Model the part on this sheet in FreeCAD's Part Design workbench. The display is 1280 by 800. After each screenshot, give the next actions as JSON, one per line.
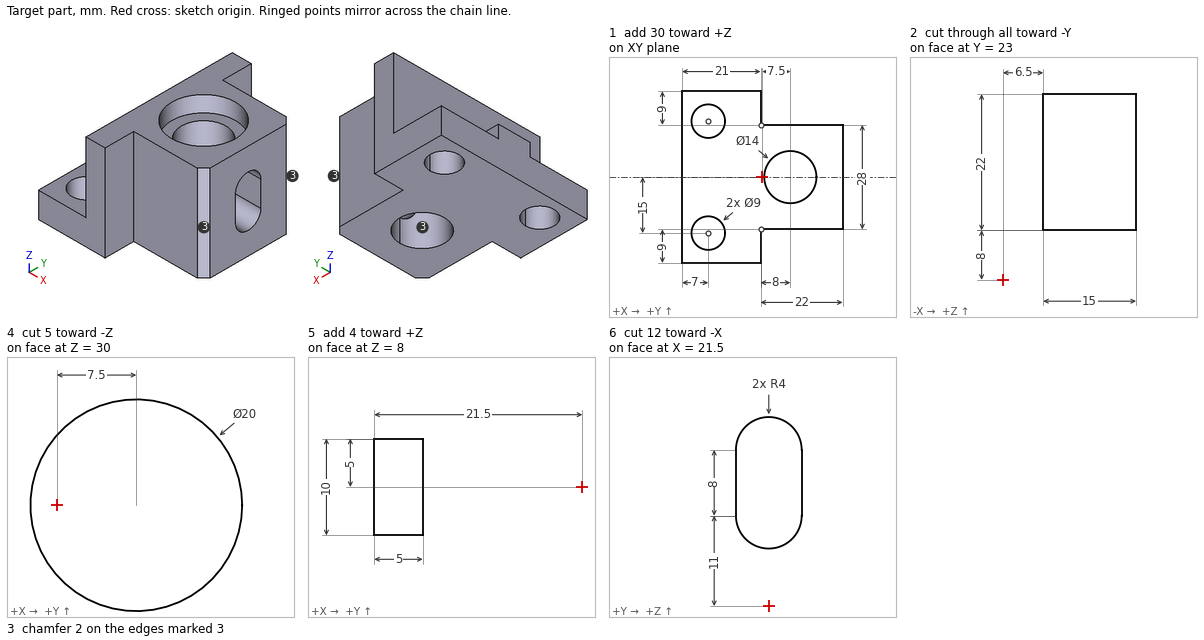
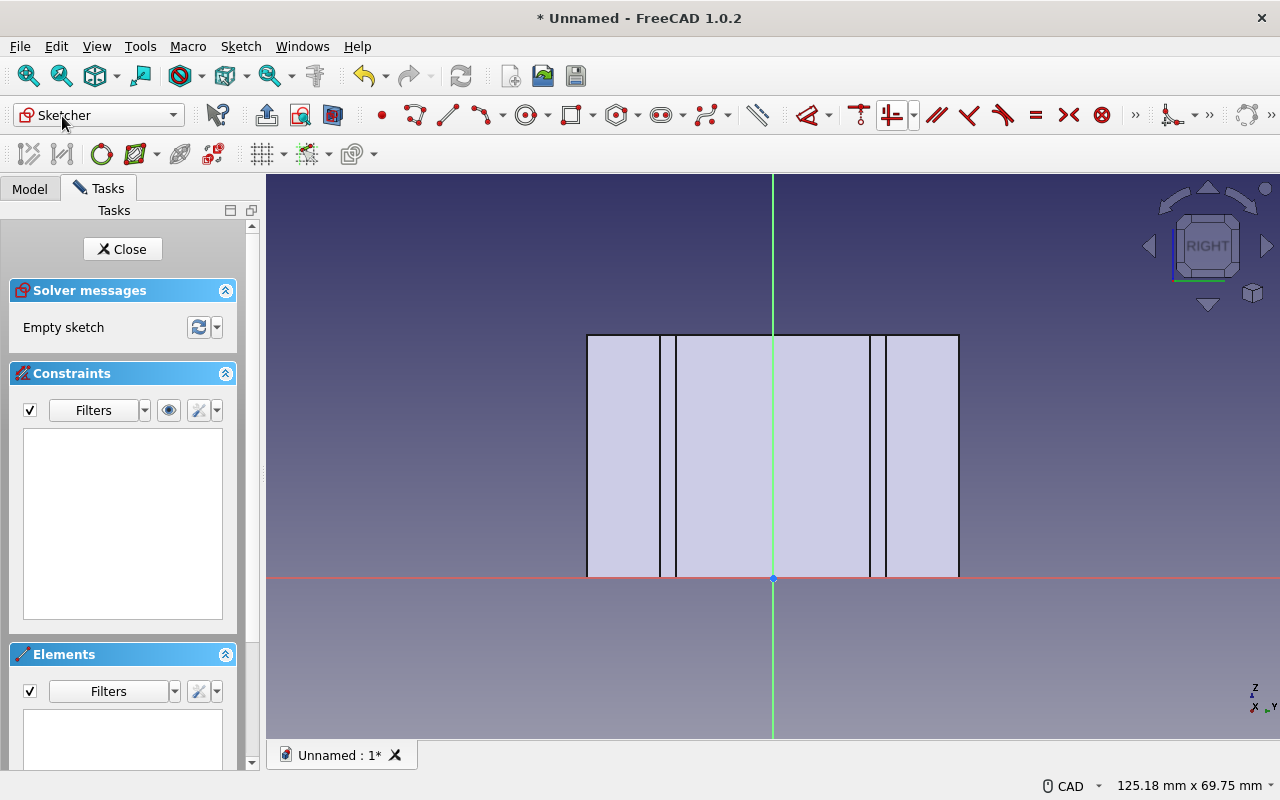
{"action": "scroll", "coordinate": [856, 519], "scroll_direction": "up", "scroll_amount": 3}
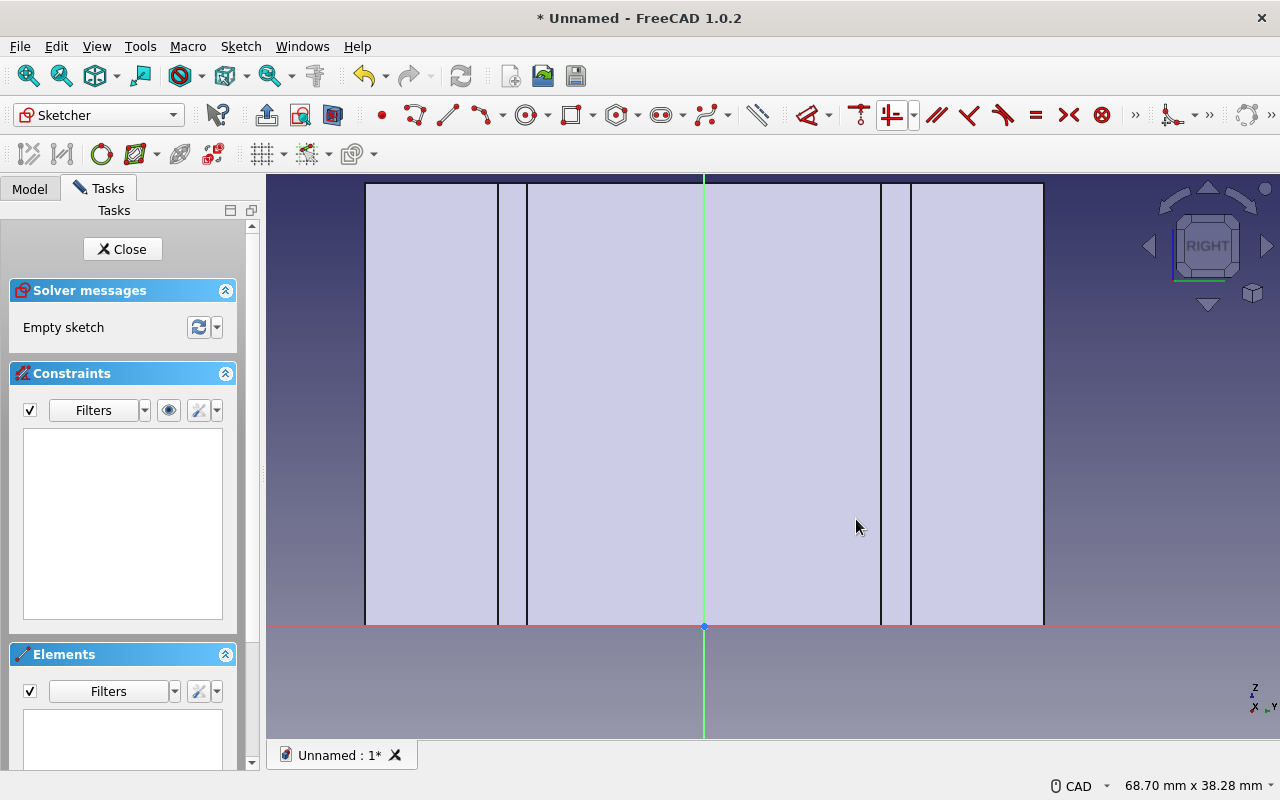
{"action": "key", "text": "g s"}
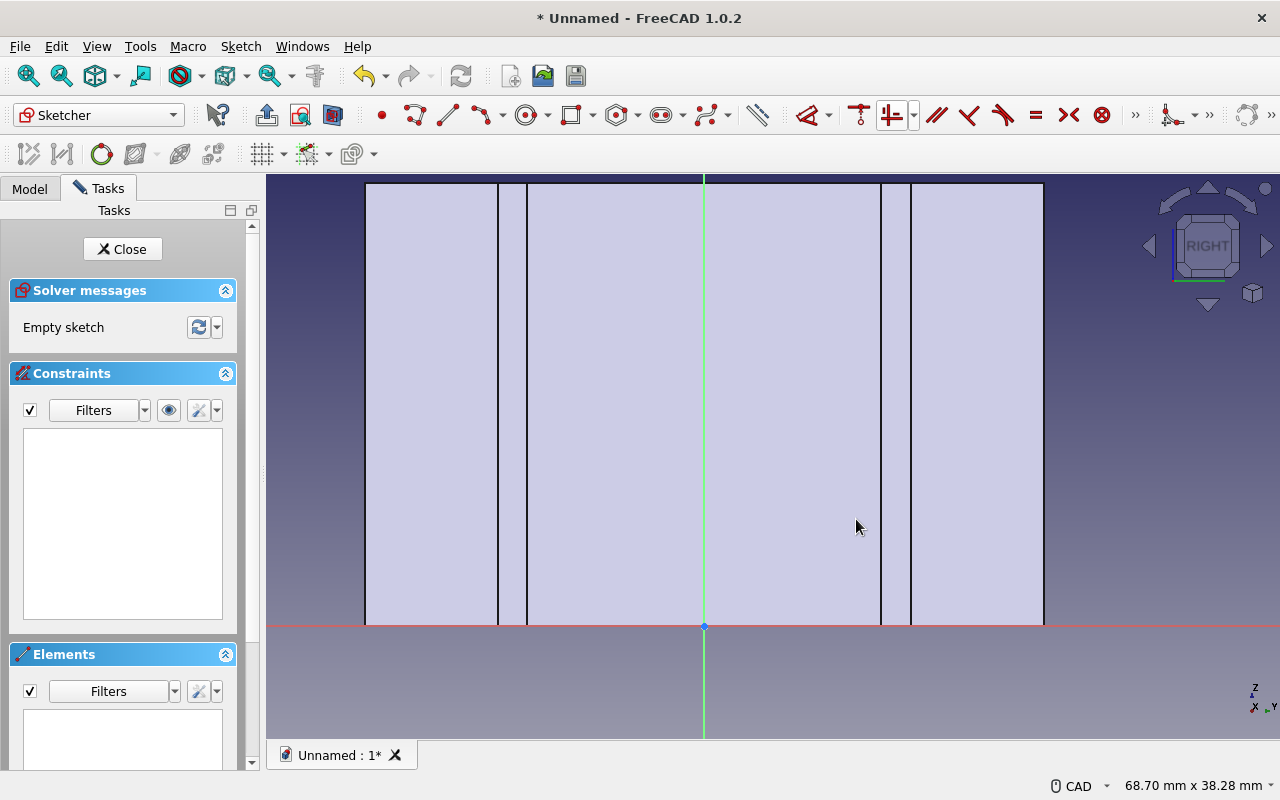
{"action": "left_click", "coordinate": [704, 464]}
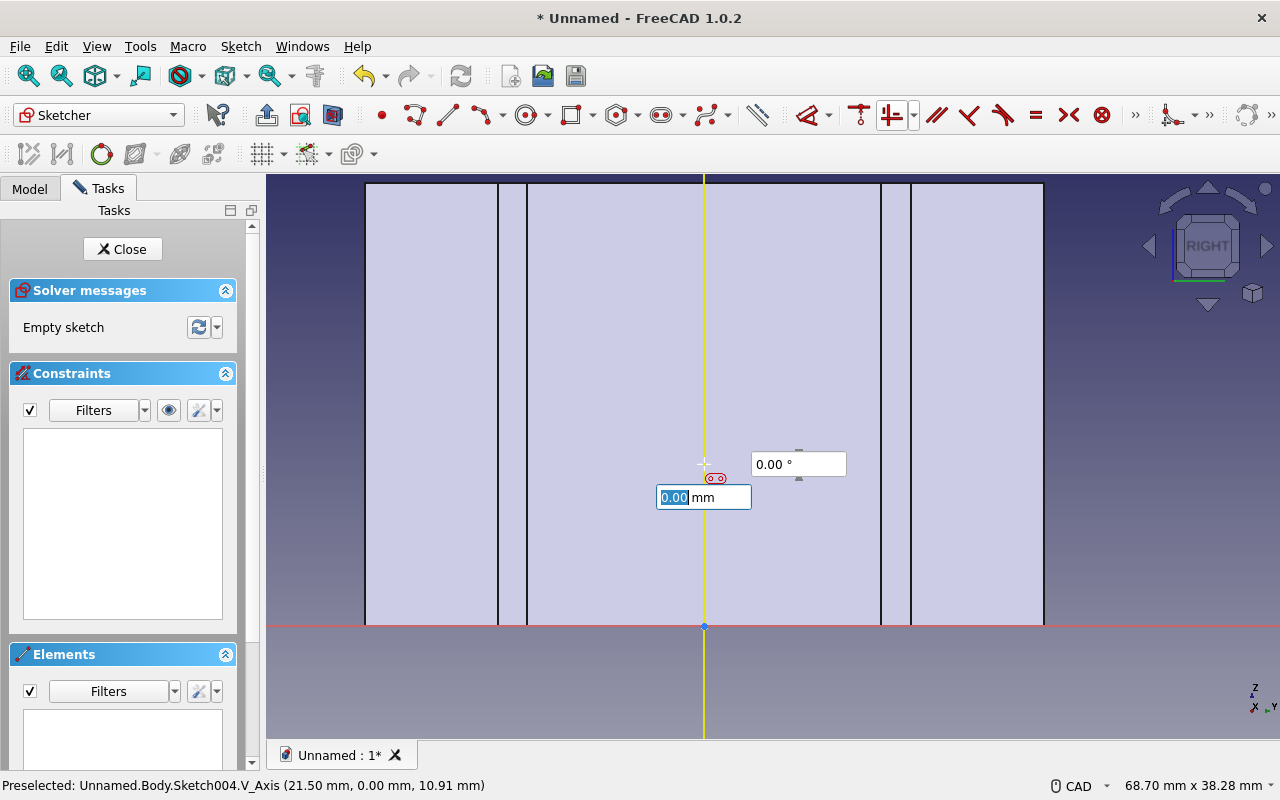
{"action": "left_click", "coordinate": [713, 346]}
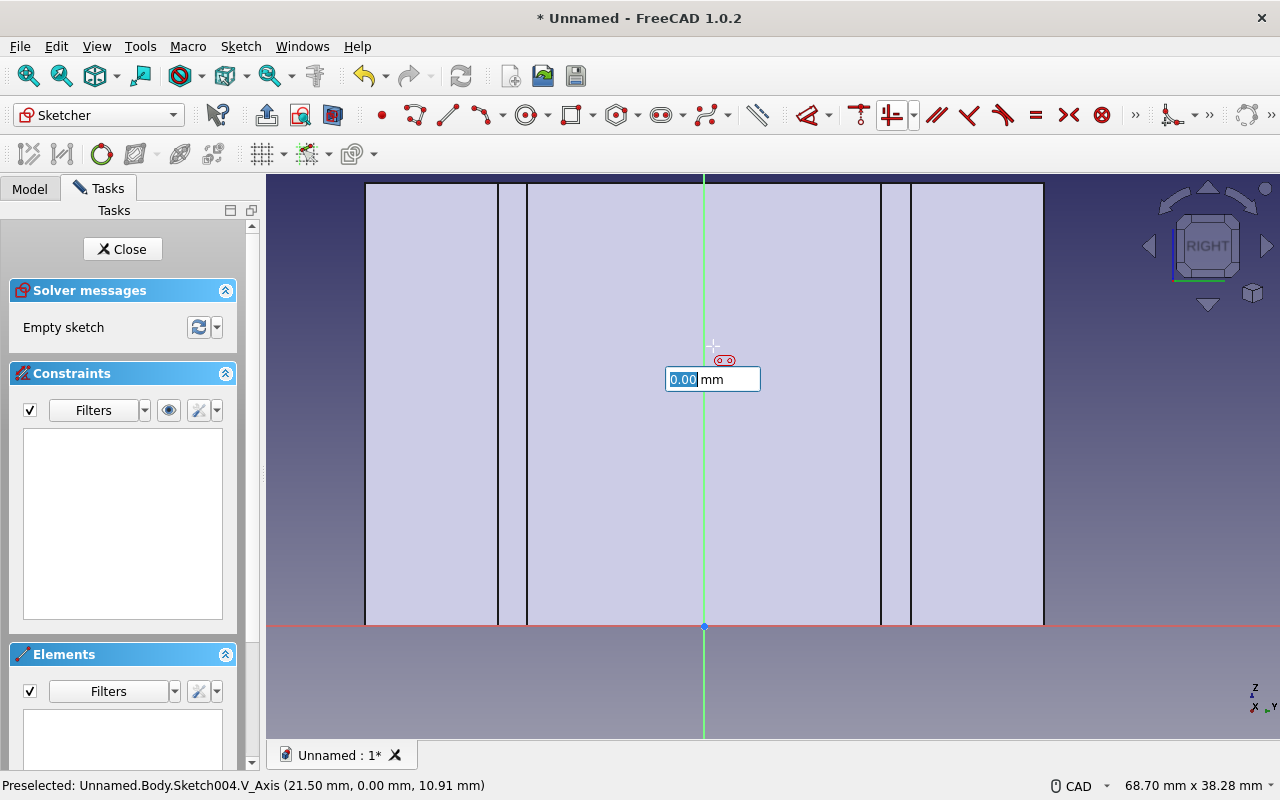
{"action": "left_click", "coordinate": [763, 405]}
{"action": "key", "text": "Escape"}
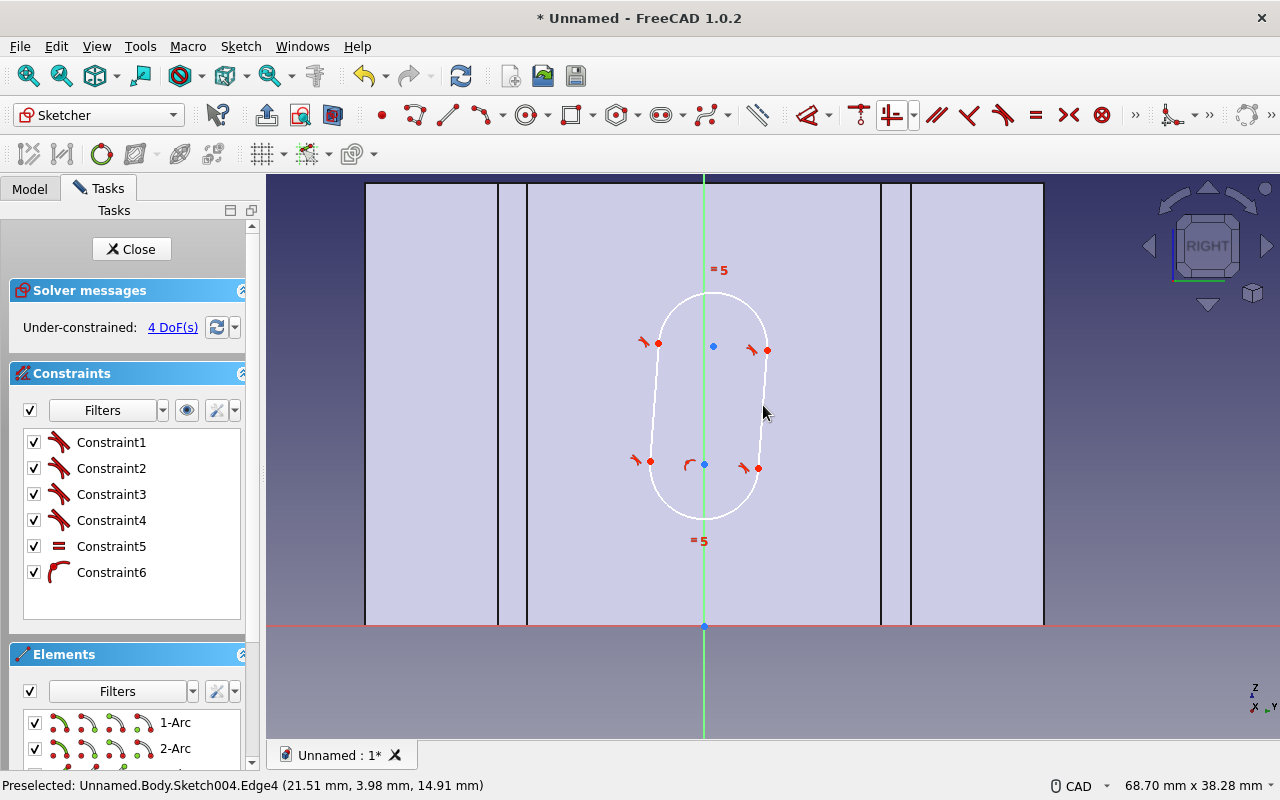
{"action": "left_click", "coordinate": [653, 426]}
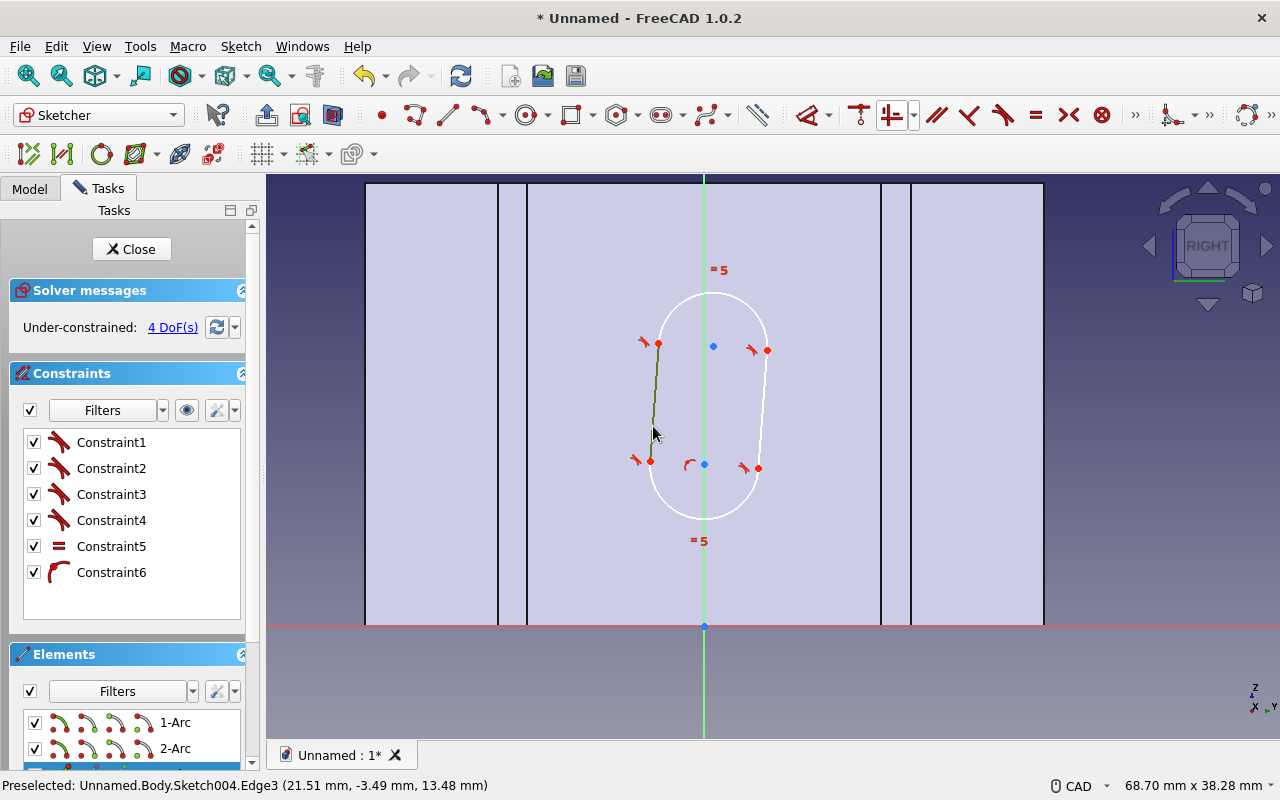
{"action": "left_click", "coordinate": [914, 116]}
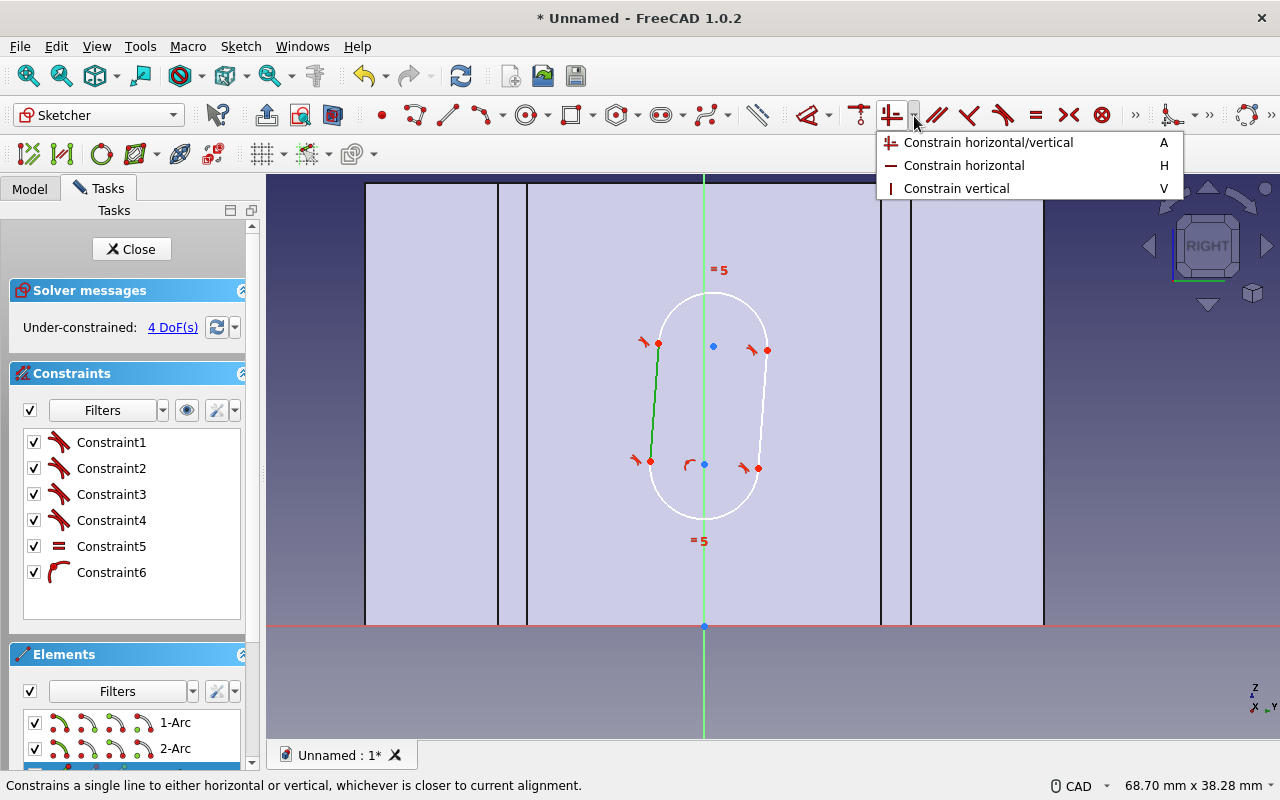
{"action": "left_click", "coordinate": [1030, 188]}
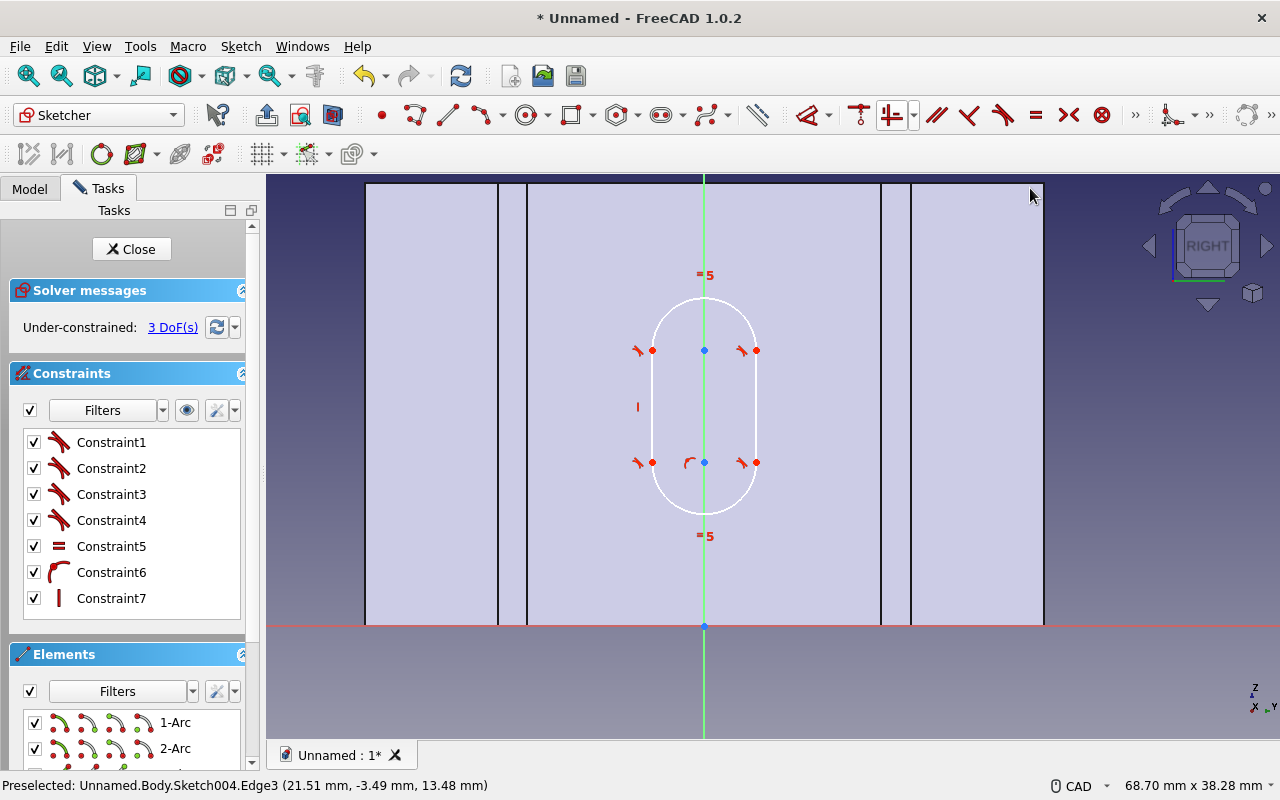
{"action": "left_click", "coordinate": [806, 116]}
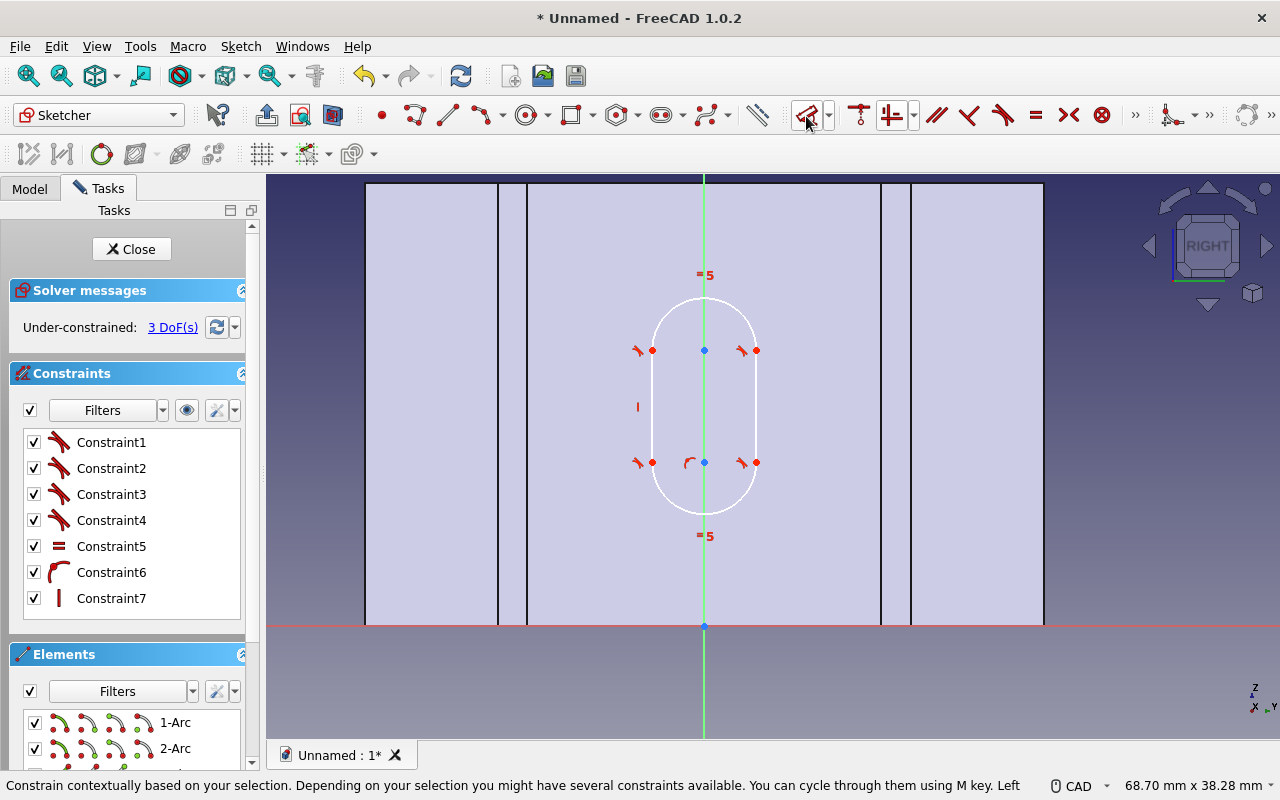
{"action": "left_click", "coordinate": [674, 504]}
{"action": "left_click", "coordinate": [655, 530]}